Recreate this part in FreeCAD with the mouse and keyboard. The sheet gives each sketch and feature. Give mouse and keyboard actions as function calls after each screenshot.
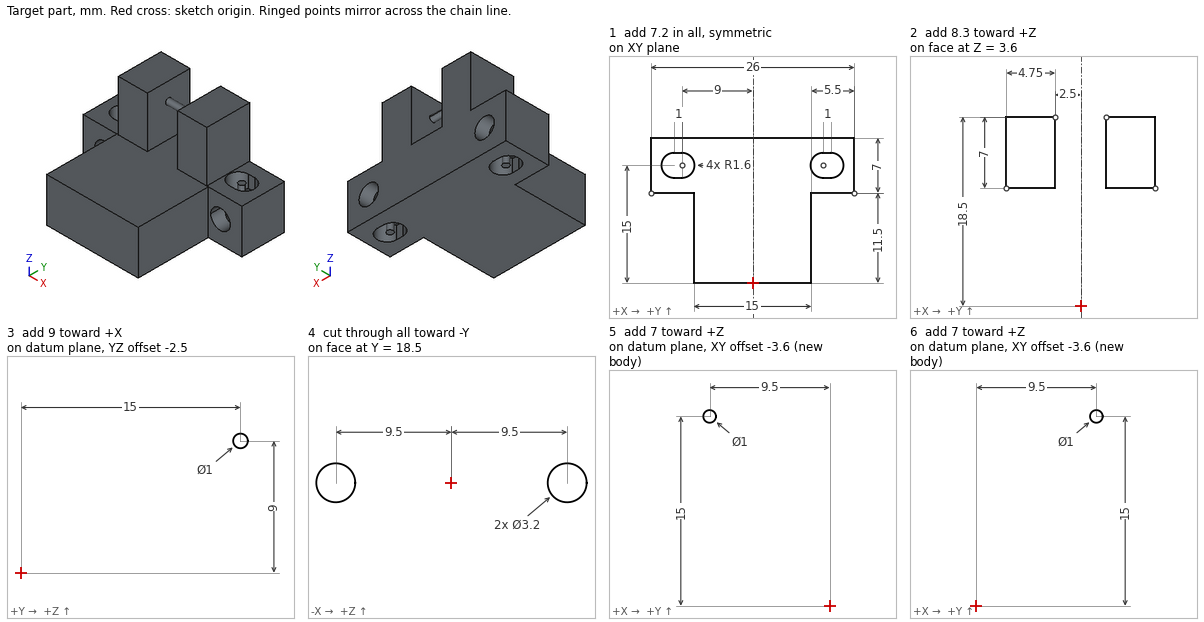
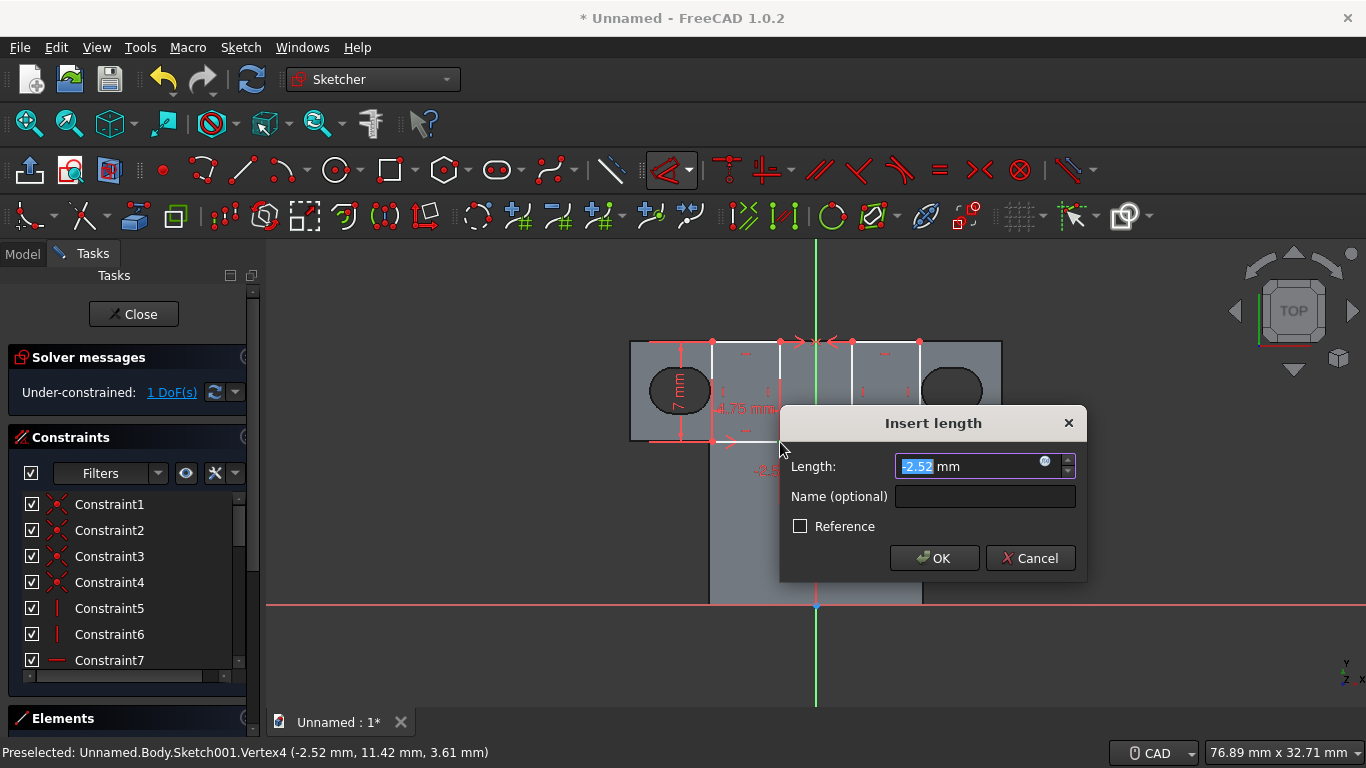
text(-2.5)
key(Return)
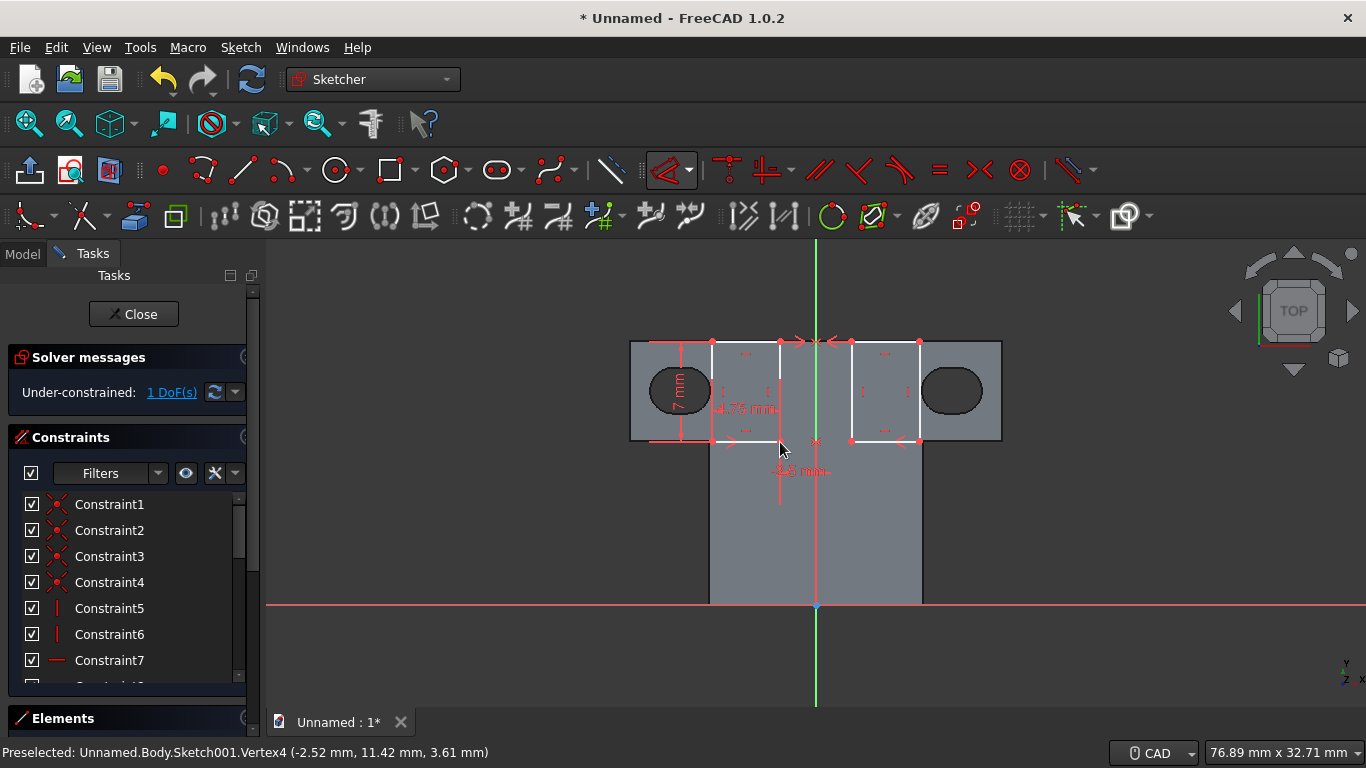
click(712, 342)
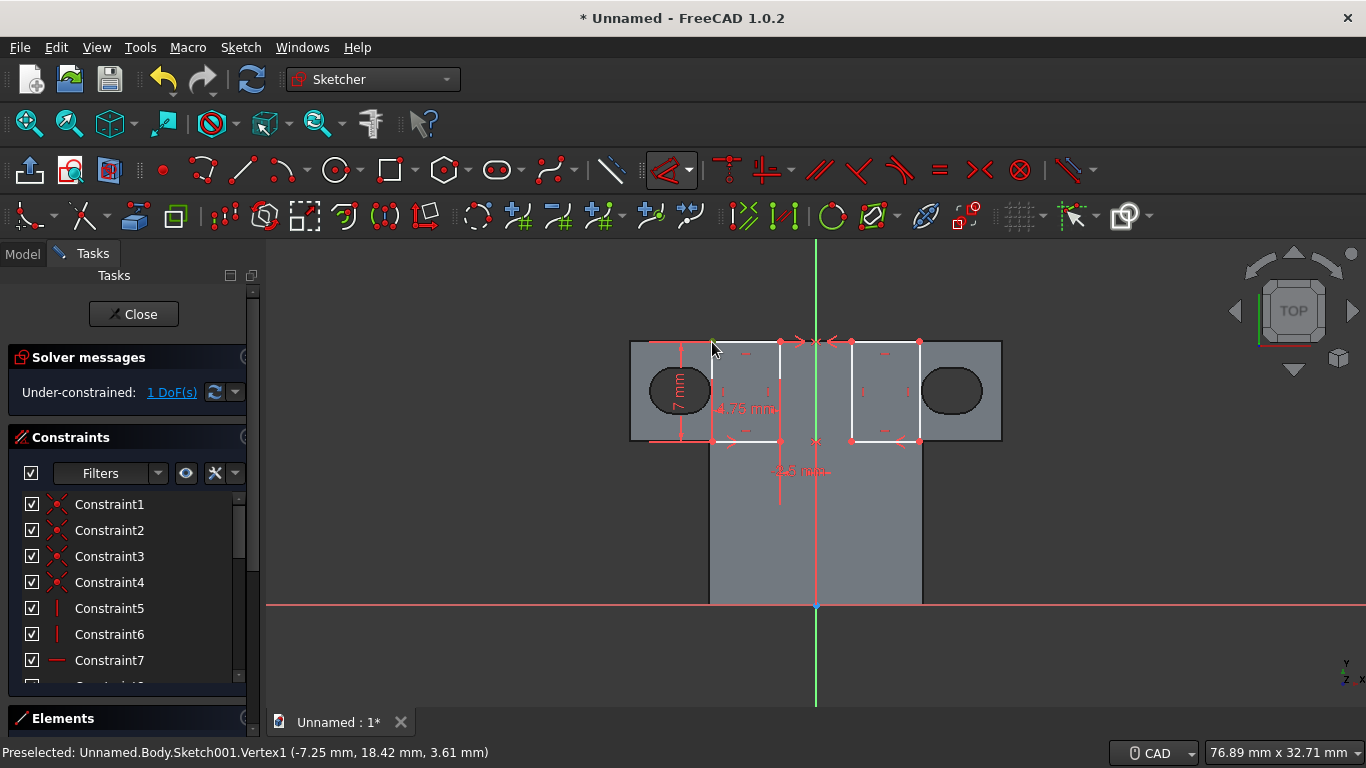
key(i)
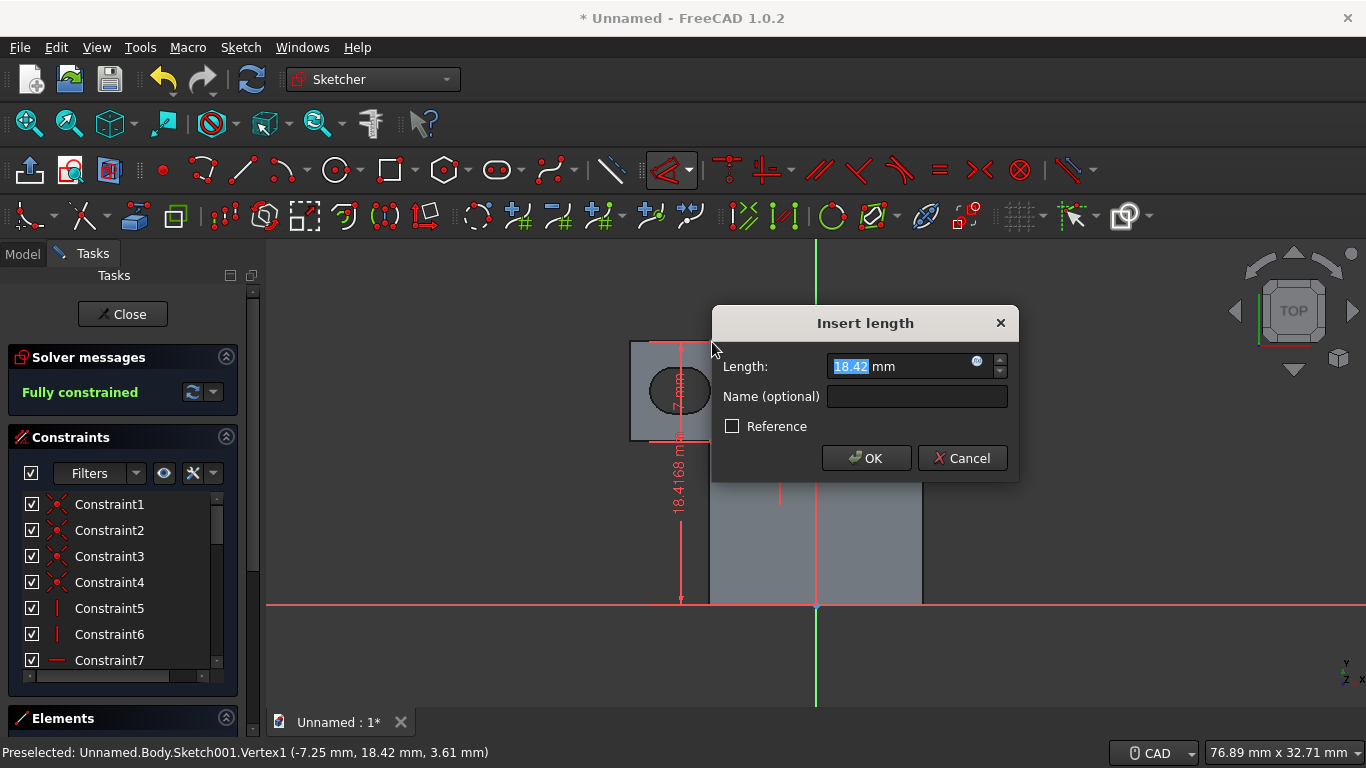
text(18.5)
key(Return)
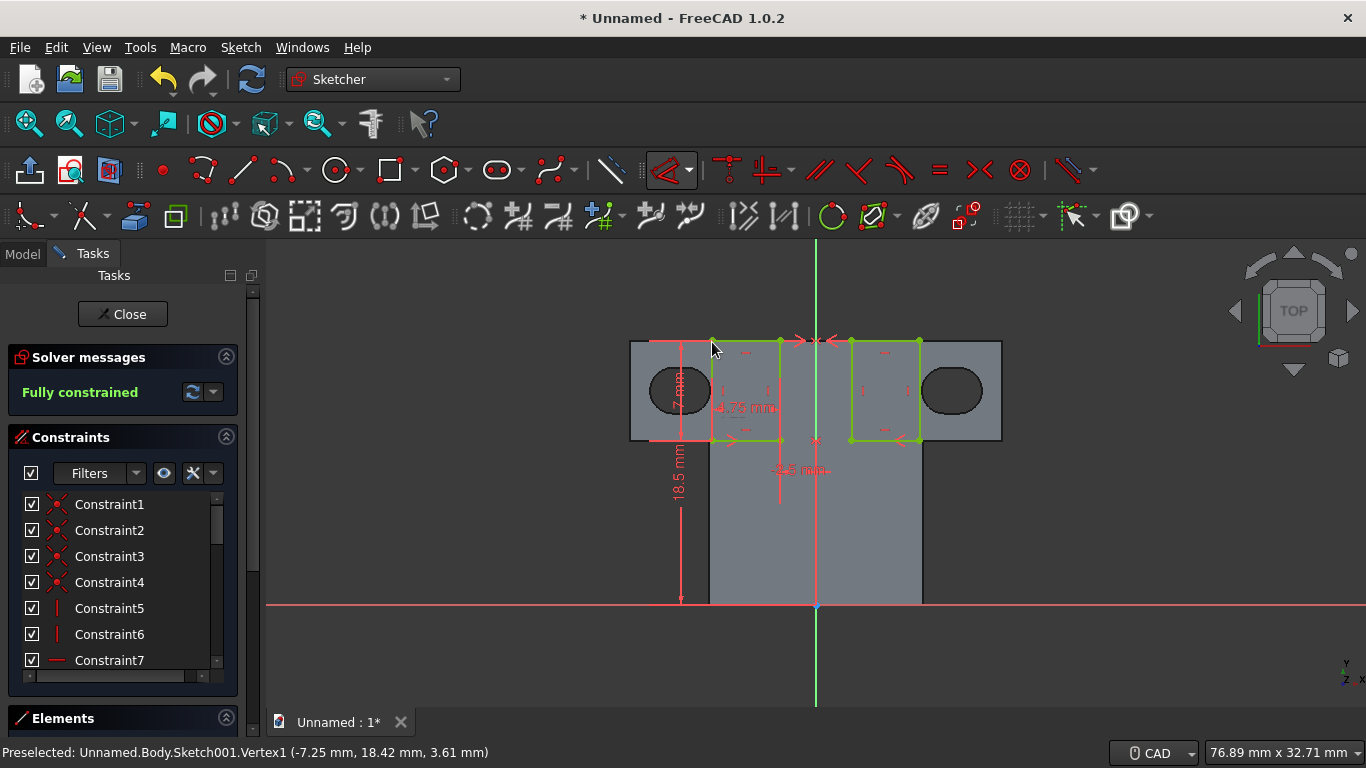
click(123, 314)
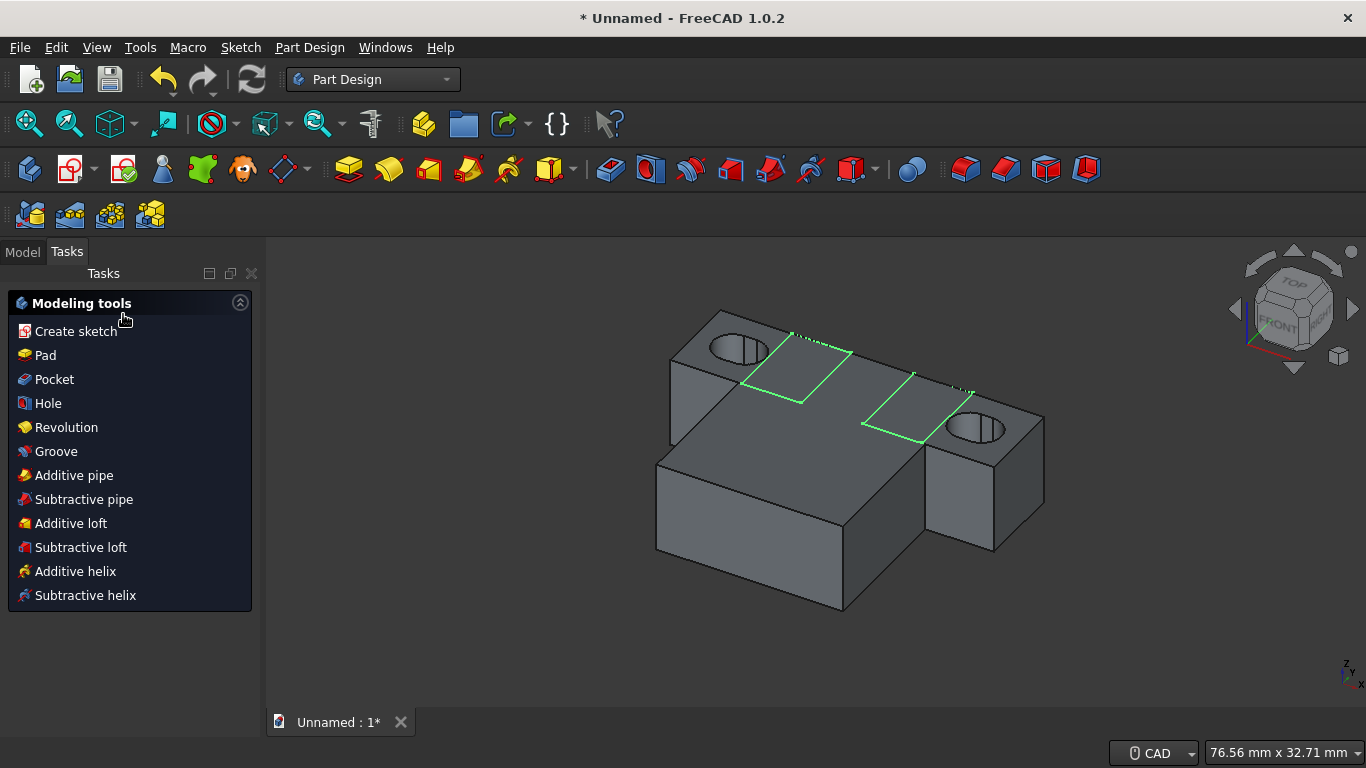
click(350, 170)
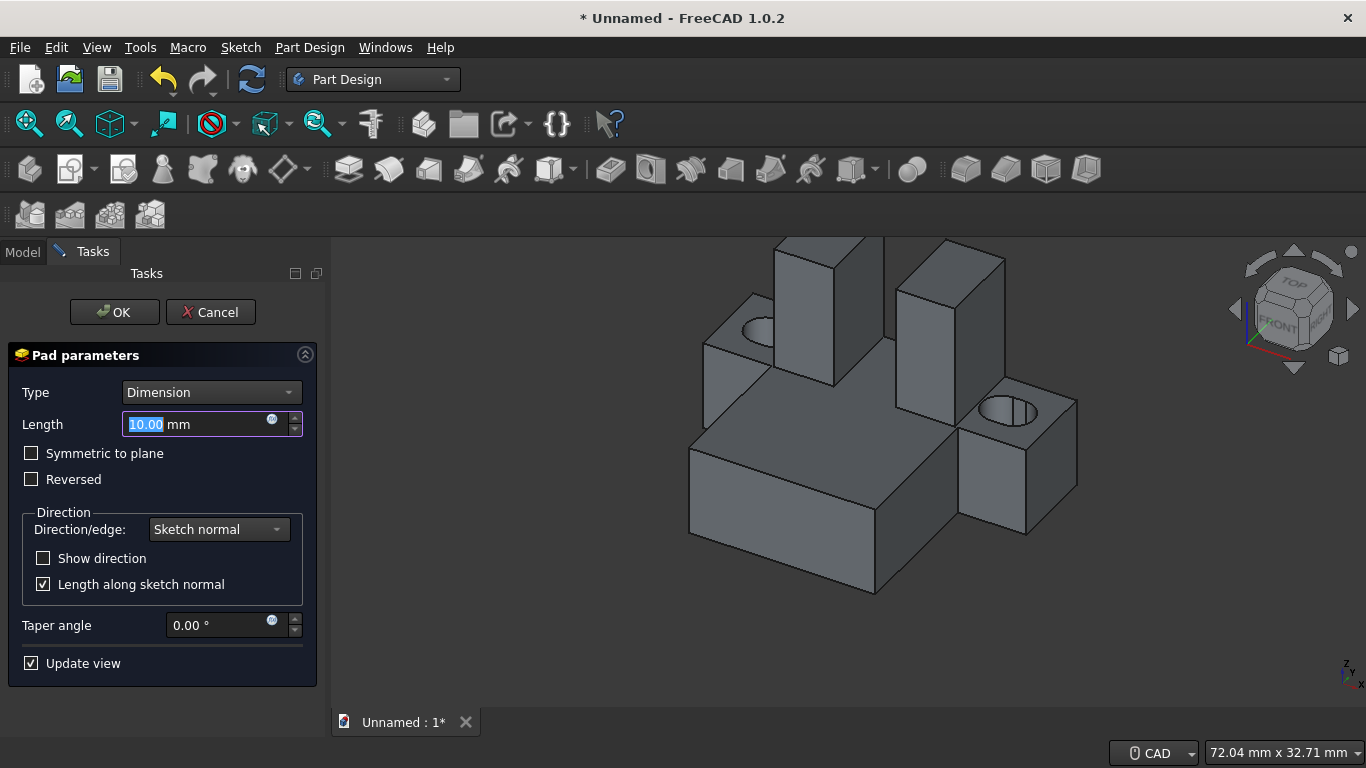
text(8.3)
key(Tab)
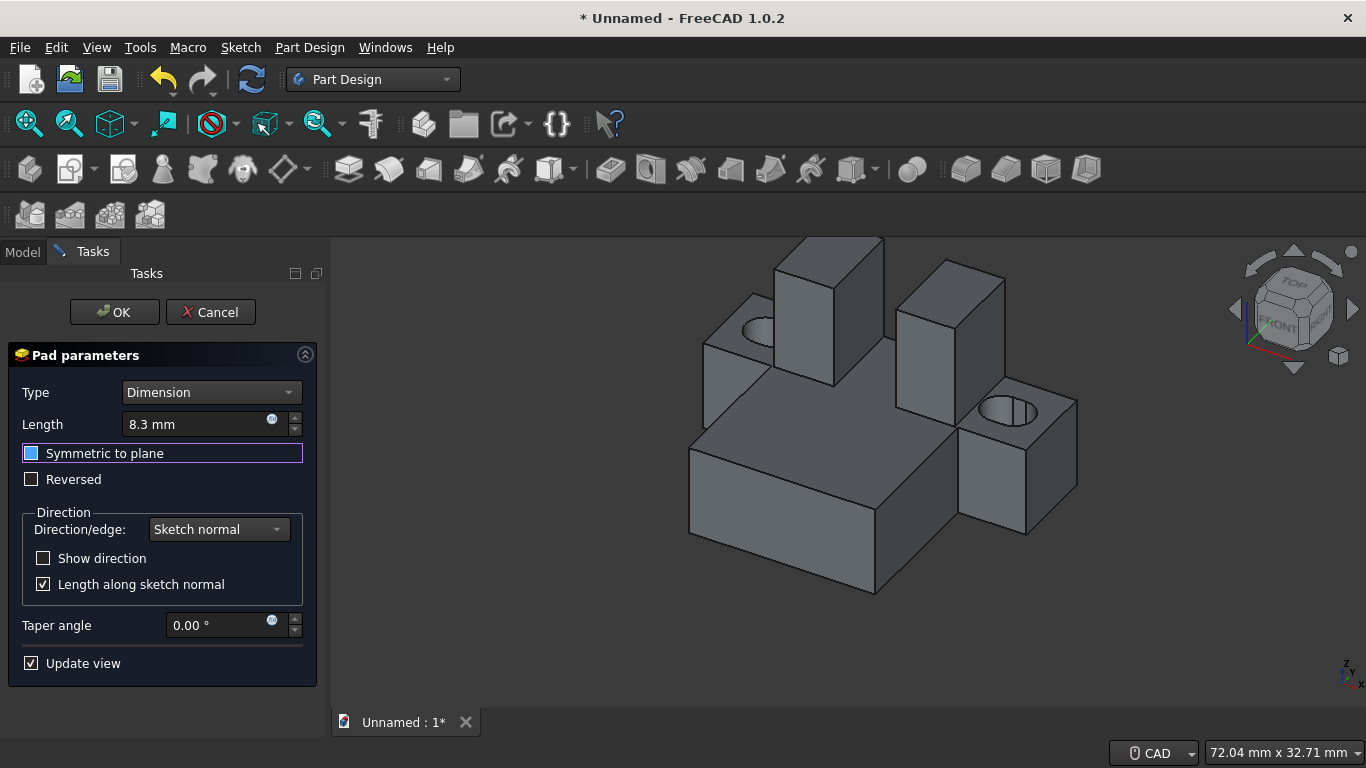
click(115, 312)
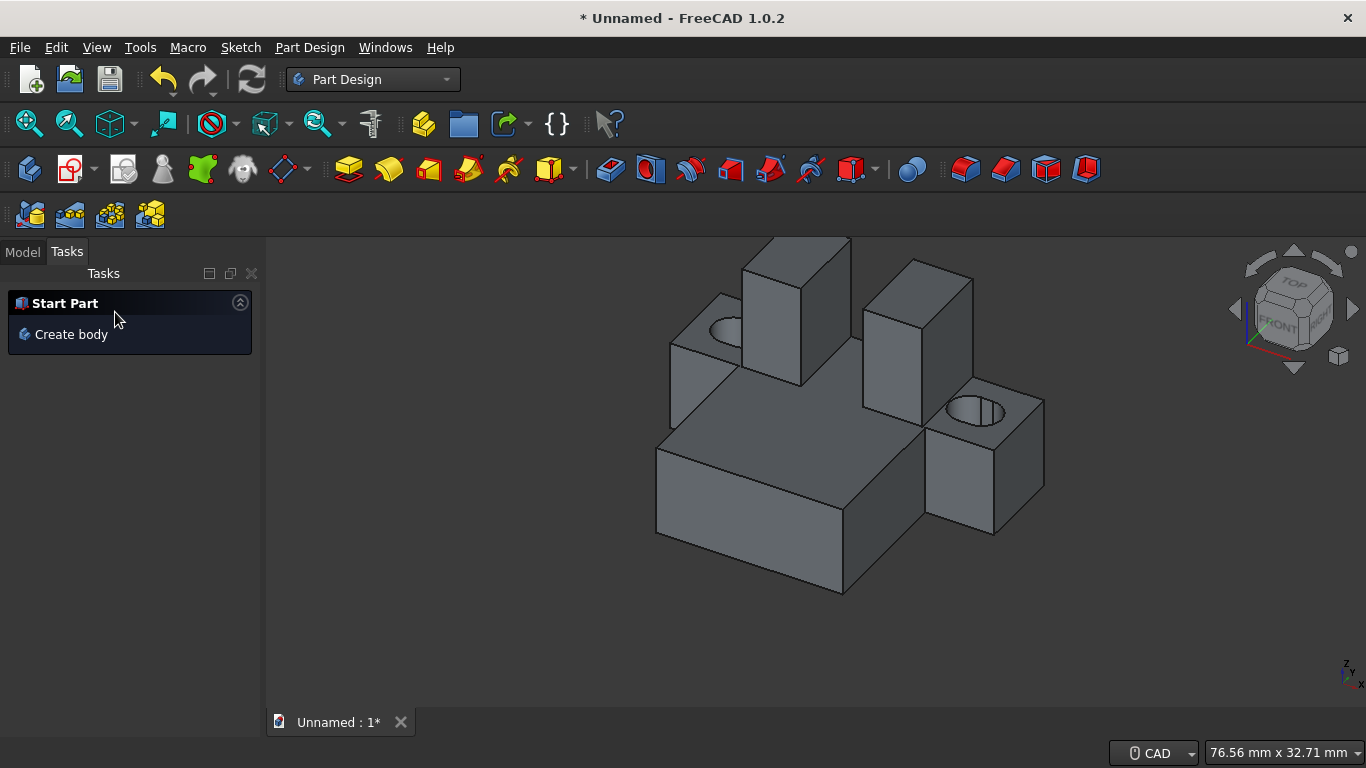
key(v)
key(f)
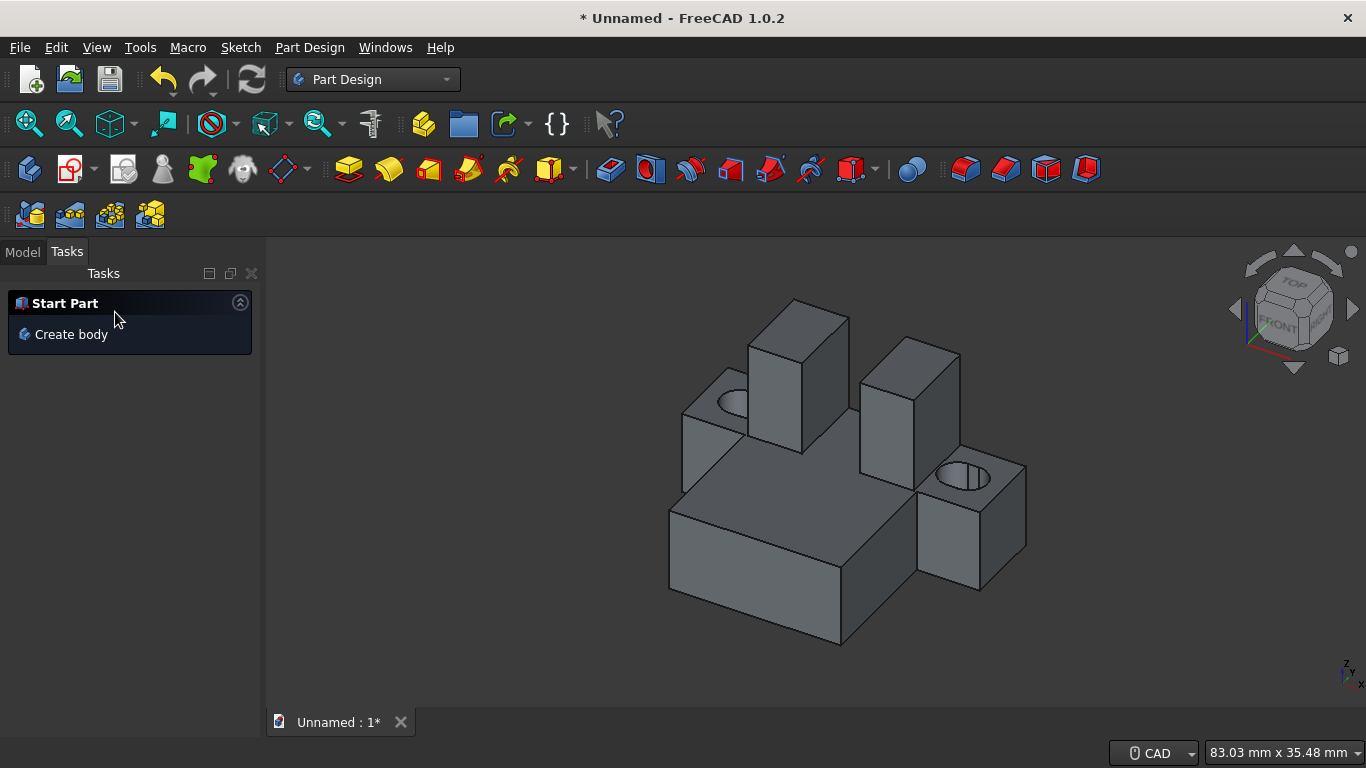
click(23, 251)